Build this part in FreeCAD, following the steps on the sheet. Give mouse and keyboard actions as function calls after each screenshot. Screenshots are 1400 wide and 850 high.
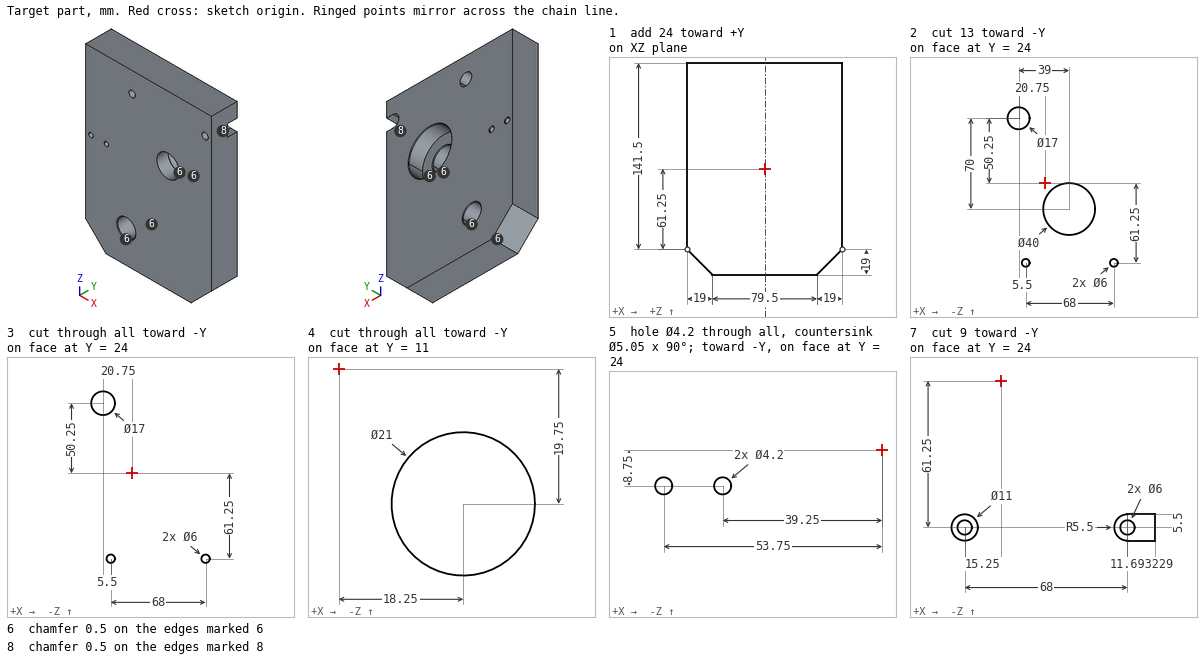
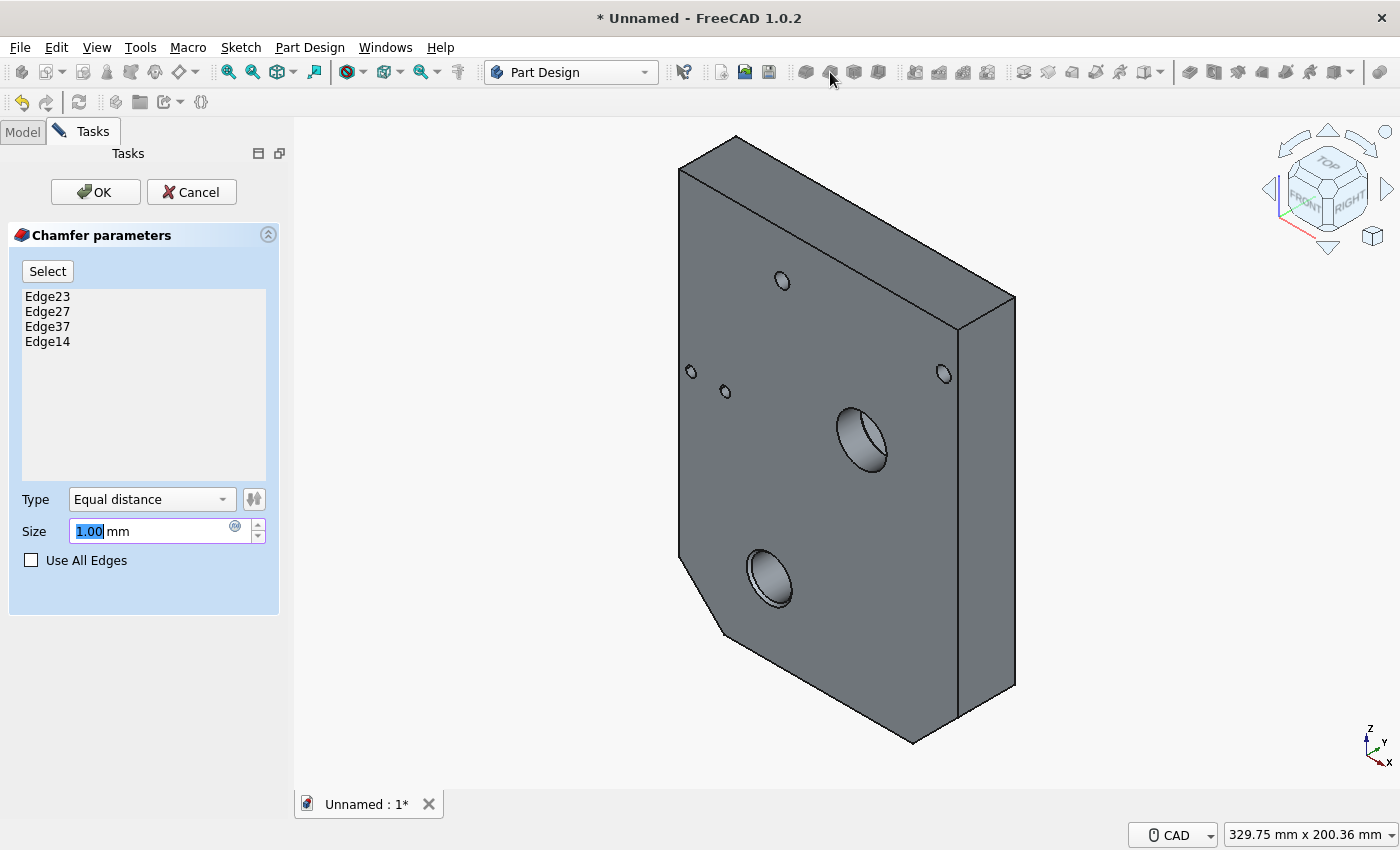
text(0.5)
key(Tab)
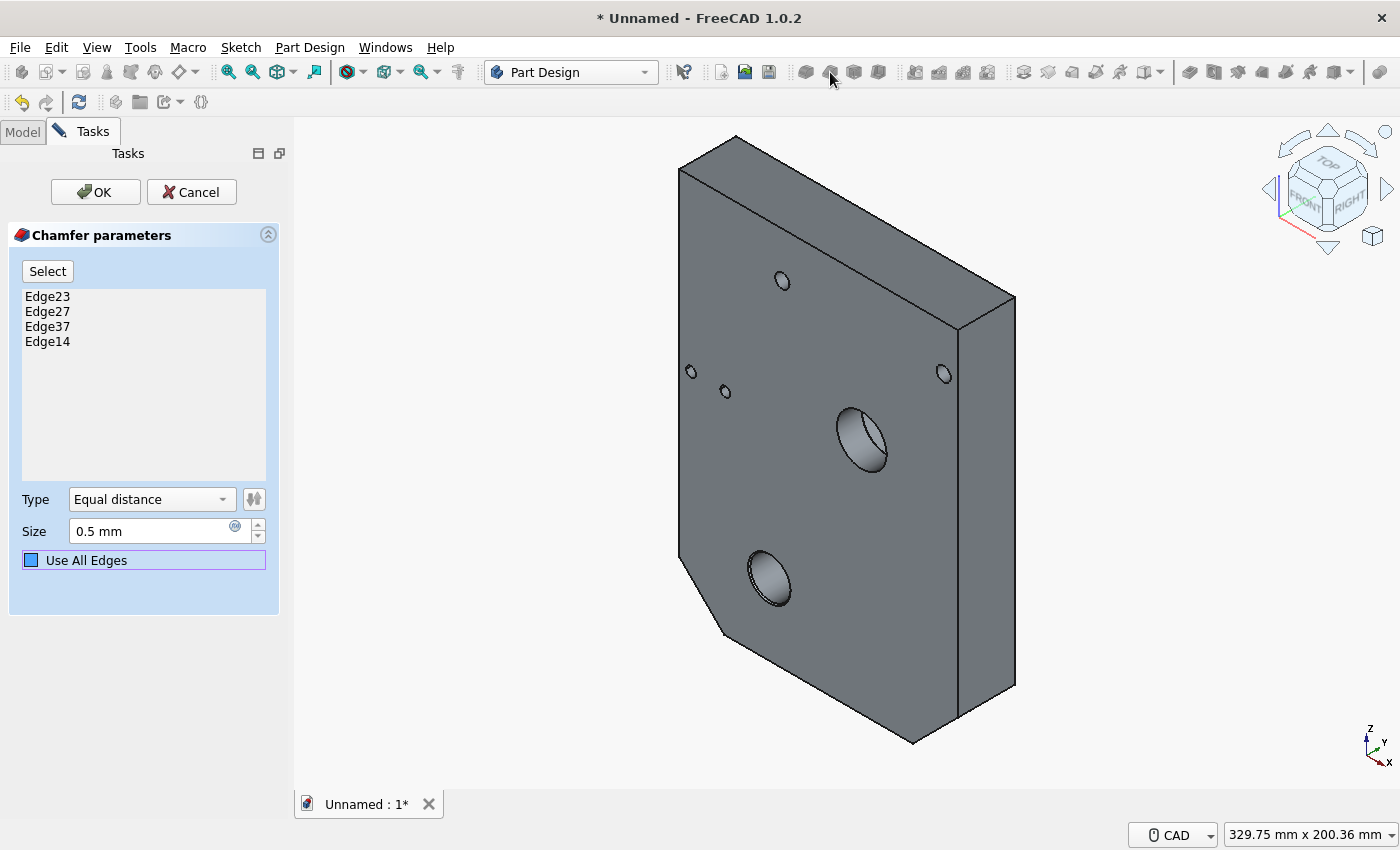
click(96, 192)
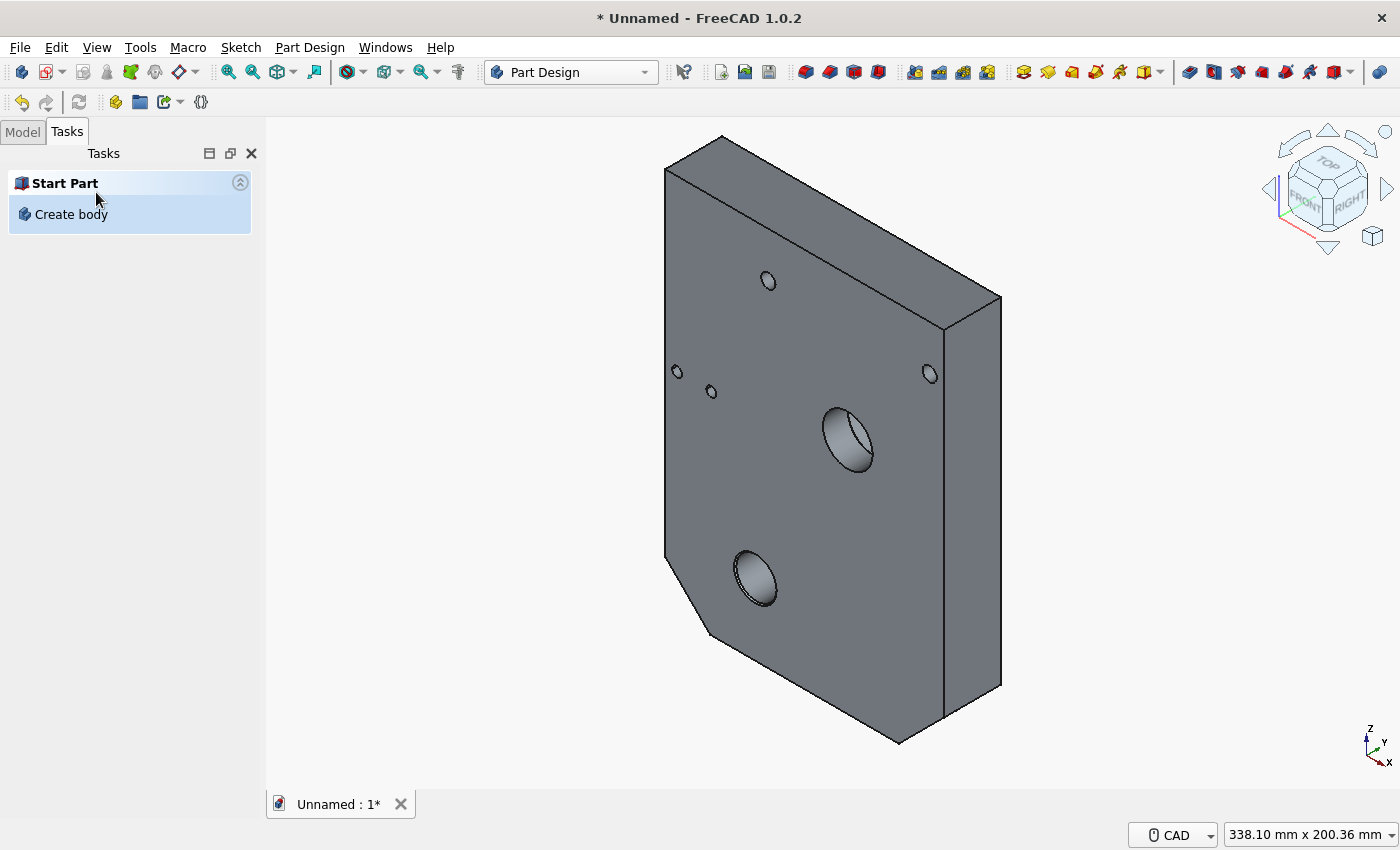
key(4)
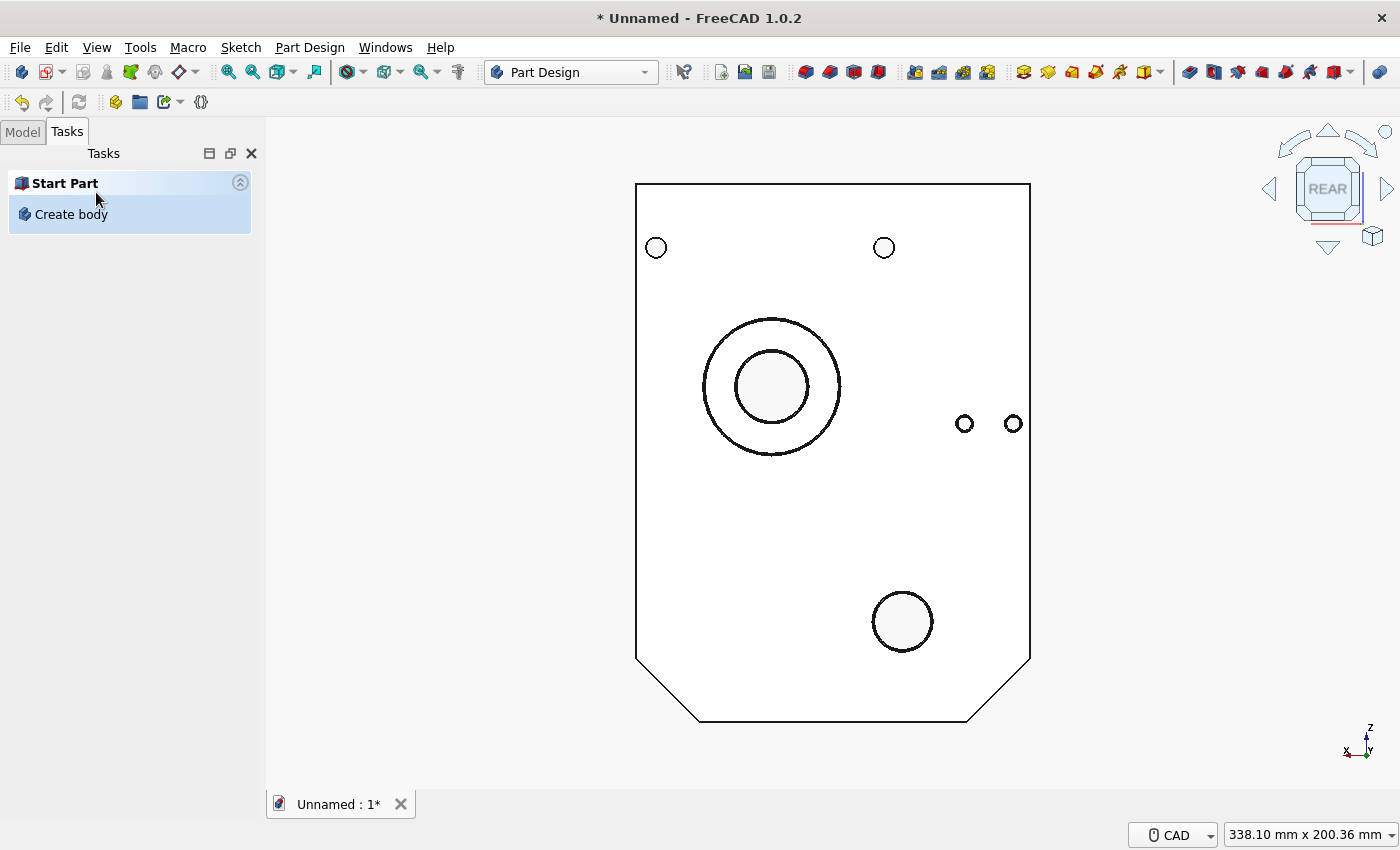
click(777, 606)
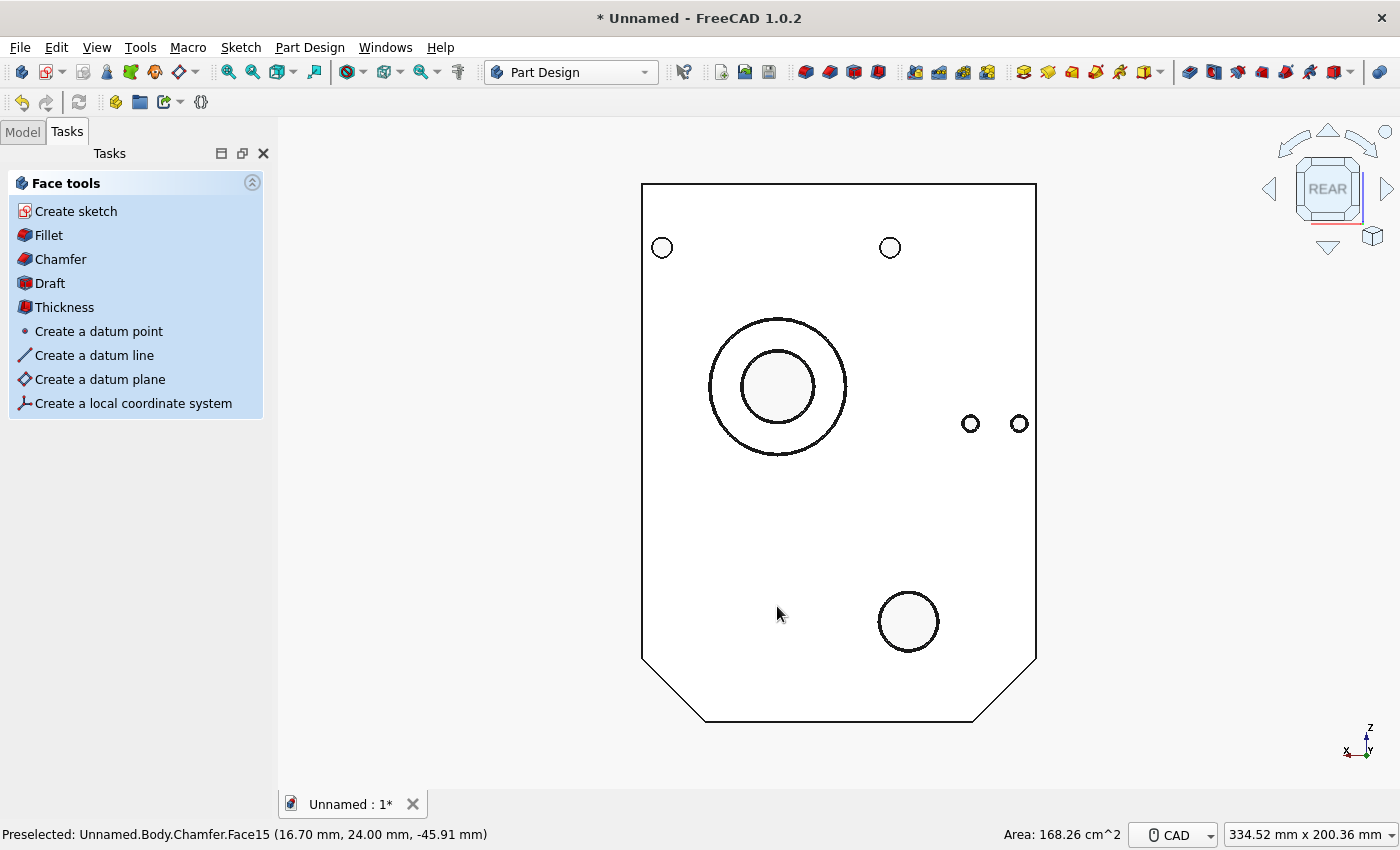
click(46, 72)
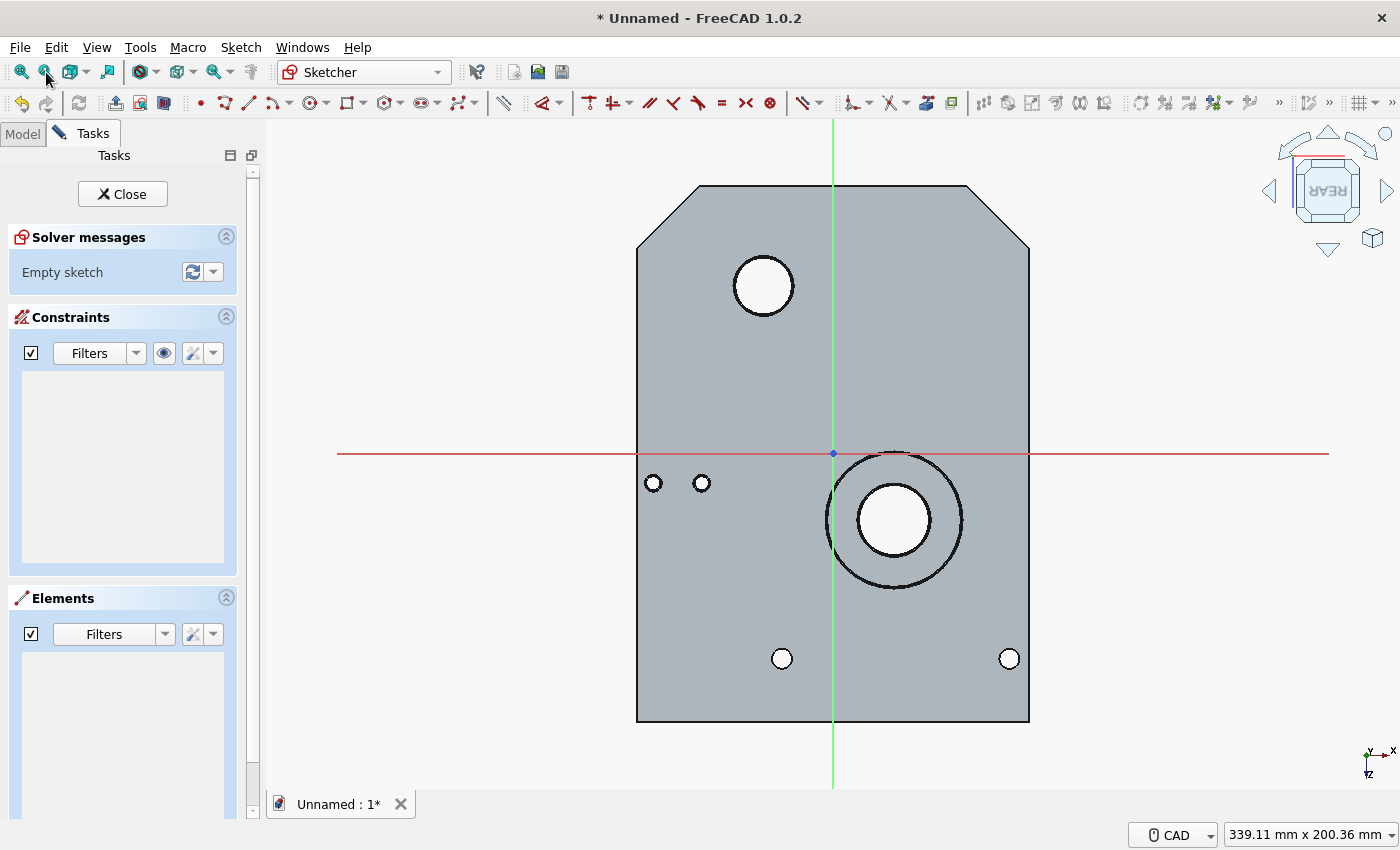
scroll(1078, 701, up, 3)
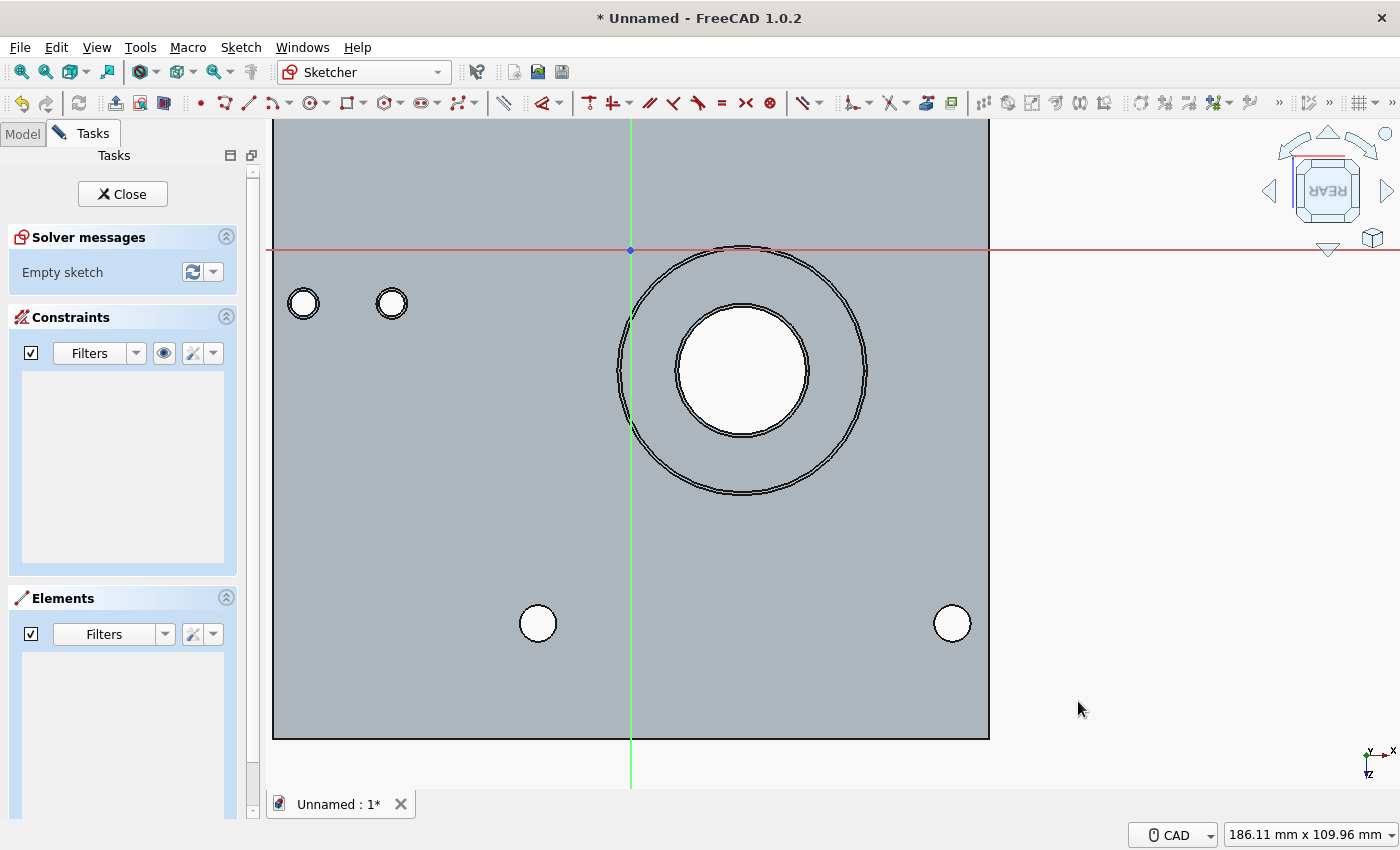
click(226, 104)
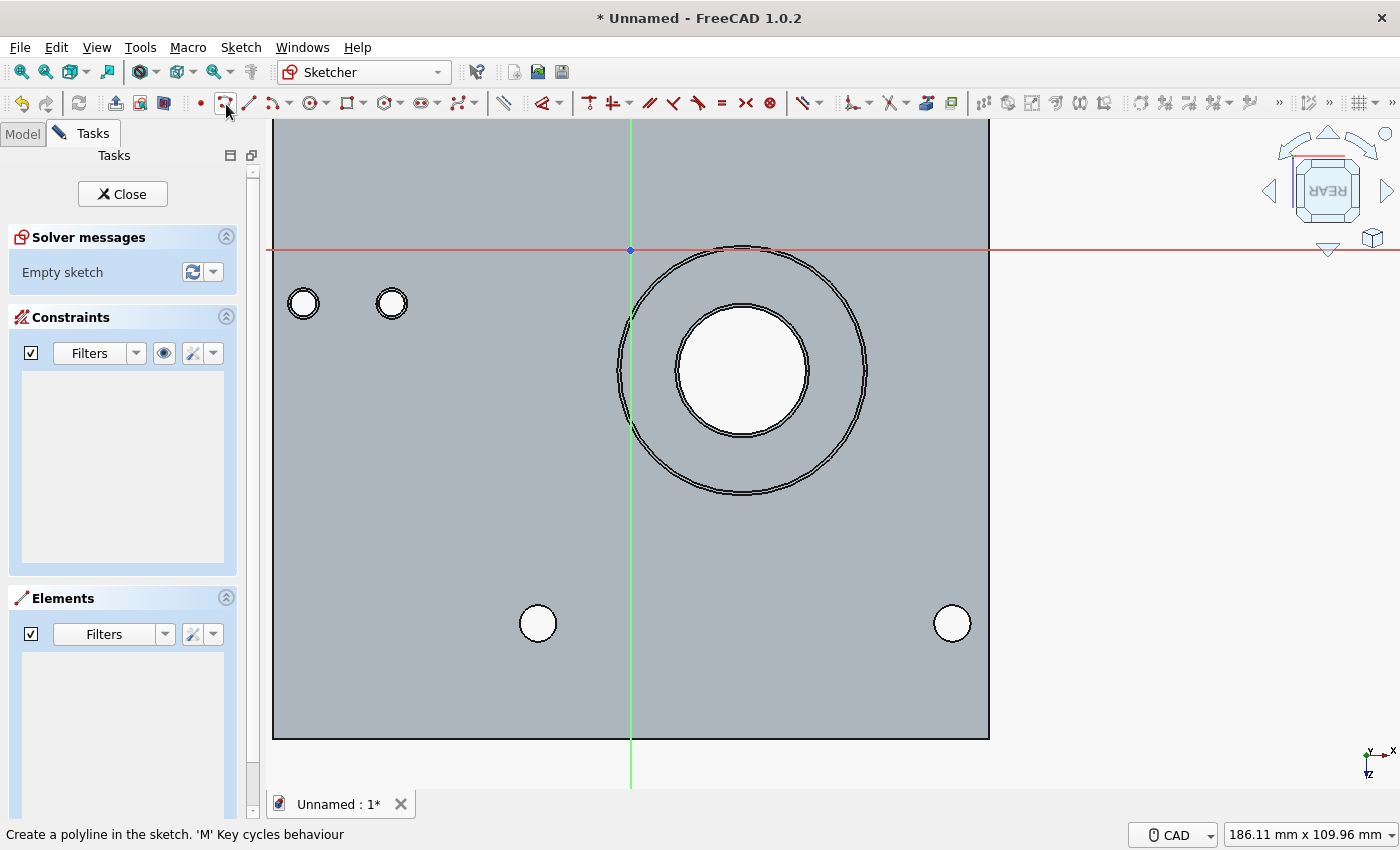
click(952, 590)
click(1024, 590)
click(1024, 657)
click(952, 657)
right_click(952, 657)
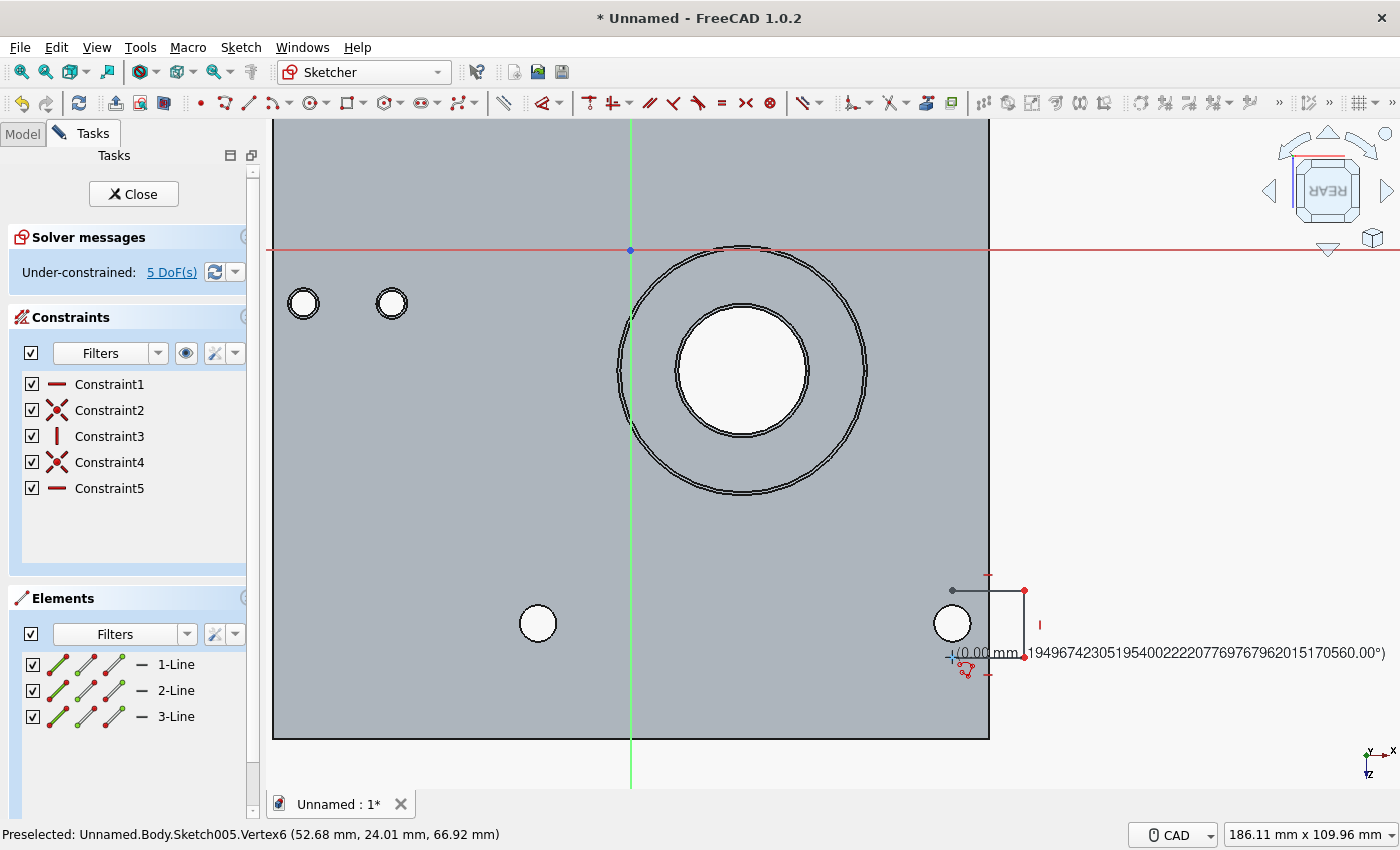
click(292, 104)